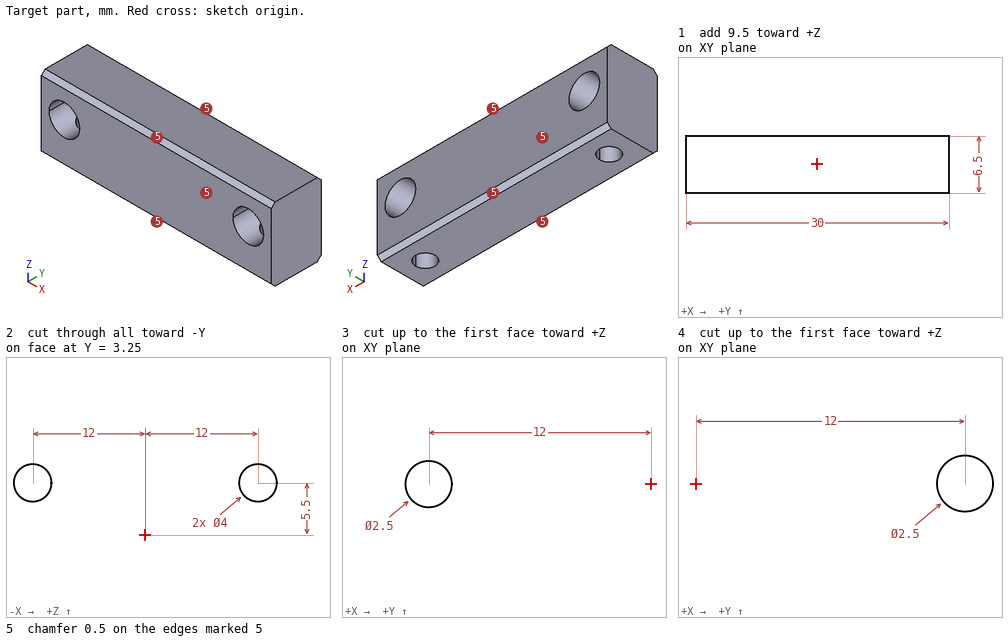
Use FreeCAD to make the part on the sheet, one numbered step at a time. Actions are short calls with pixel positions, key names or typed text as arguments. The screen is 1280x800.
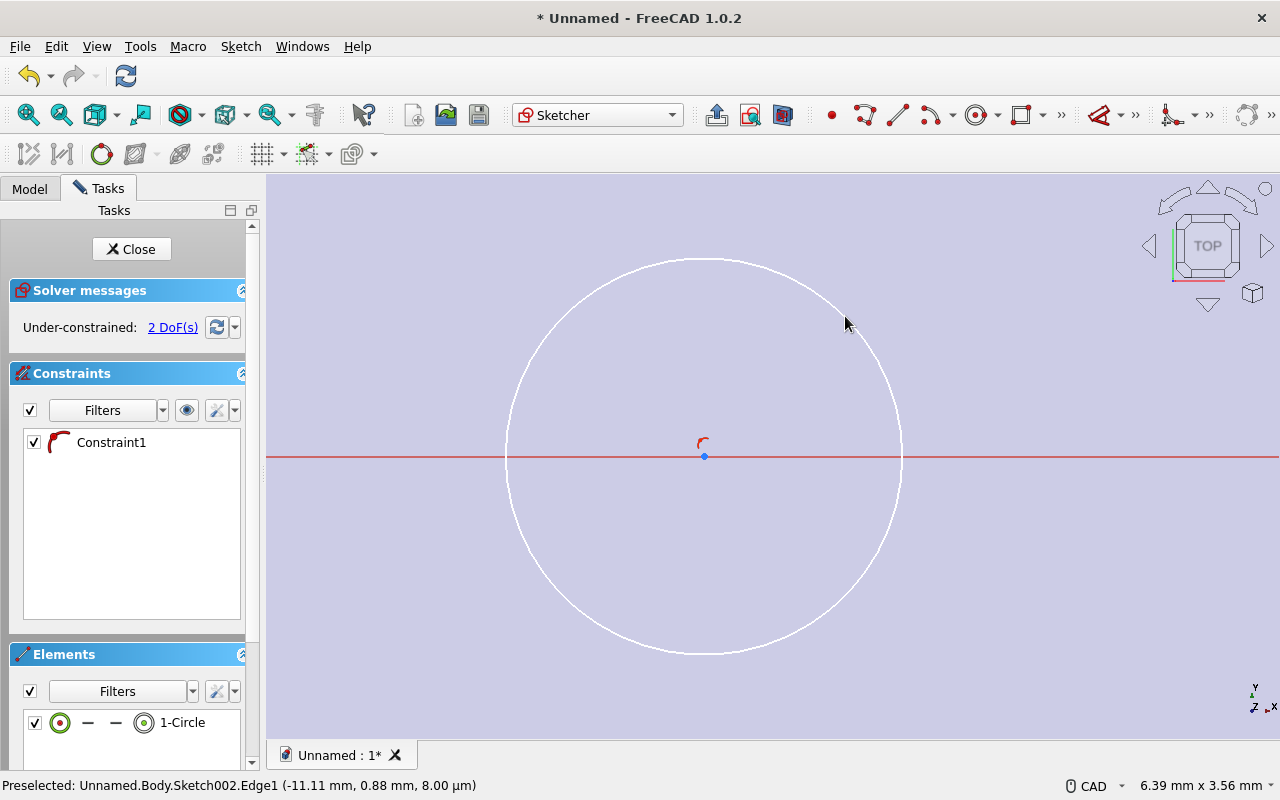
key(d)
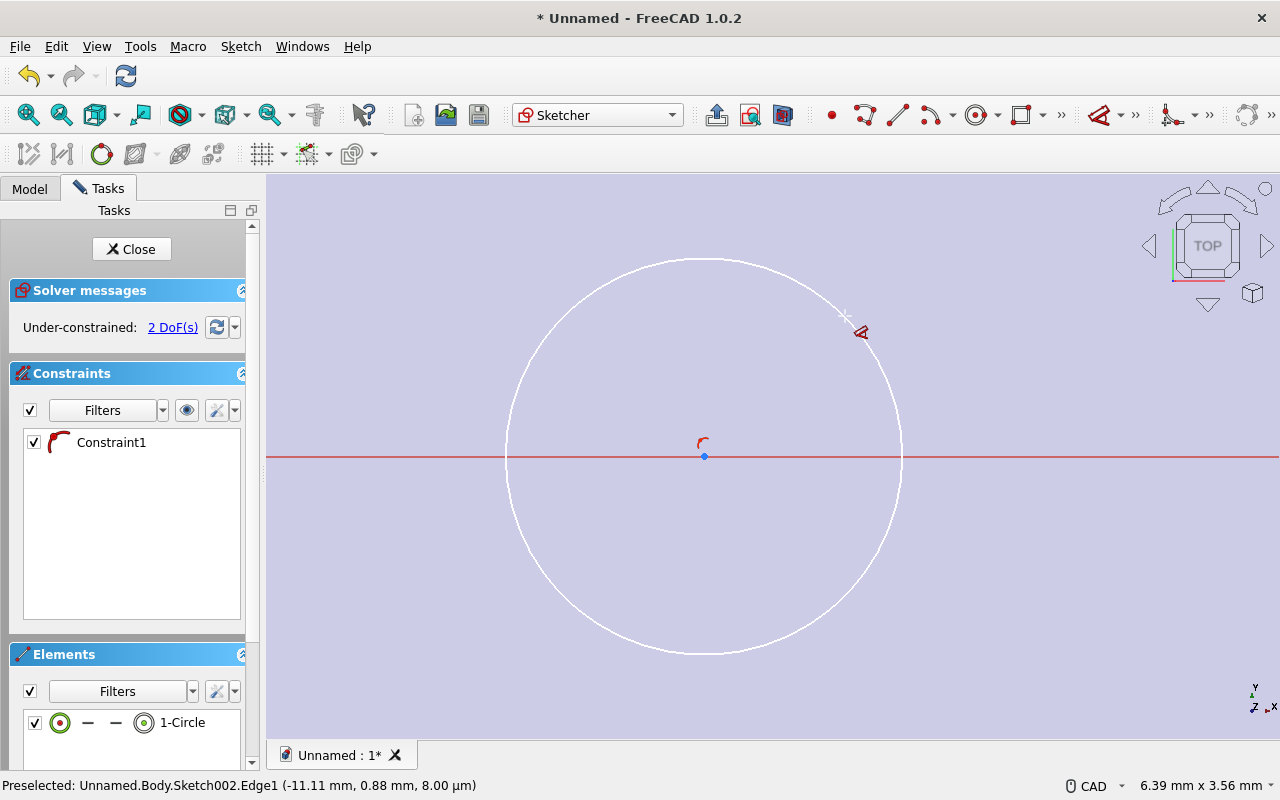
click(844, 316)
click(867, 293)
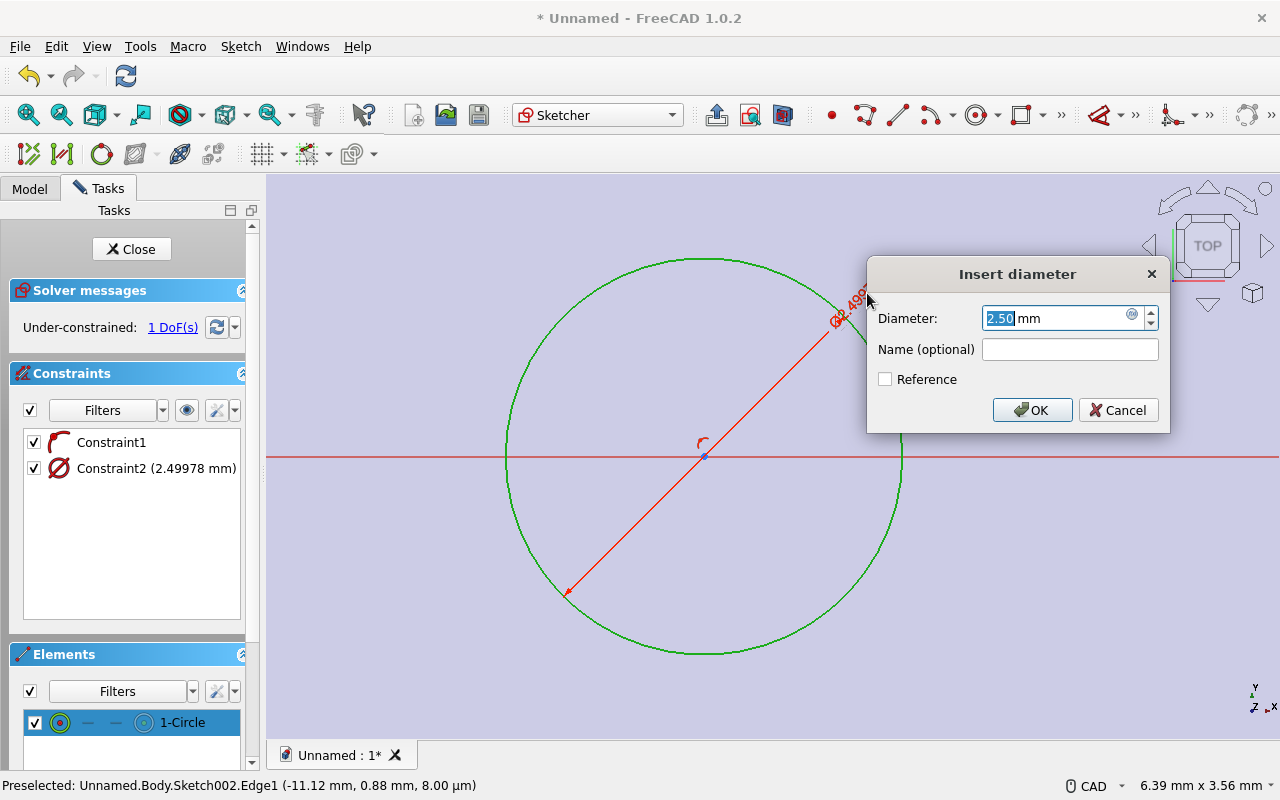
text(2.5)
key(Return)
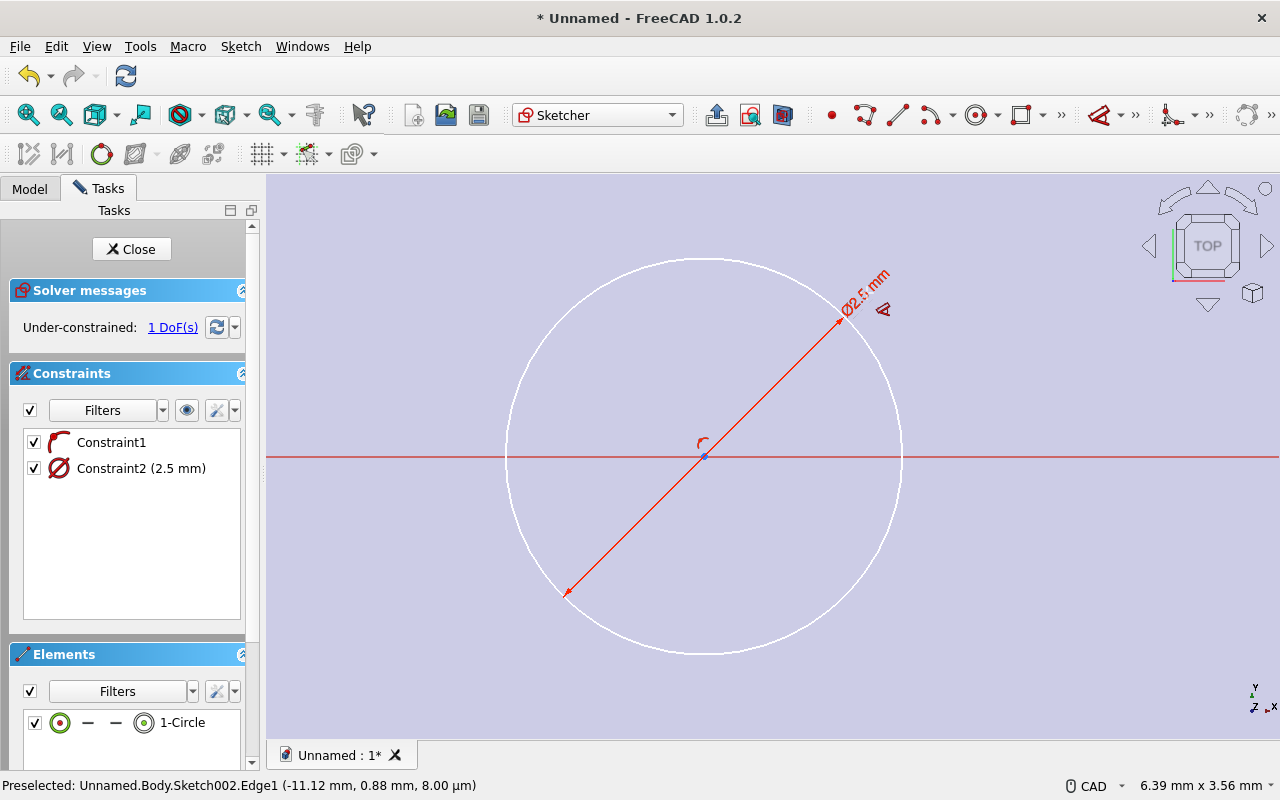
click(704, 456)
click(815, 490)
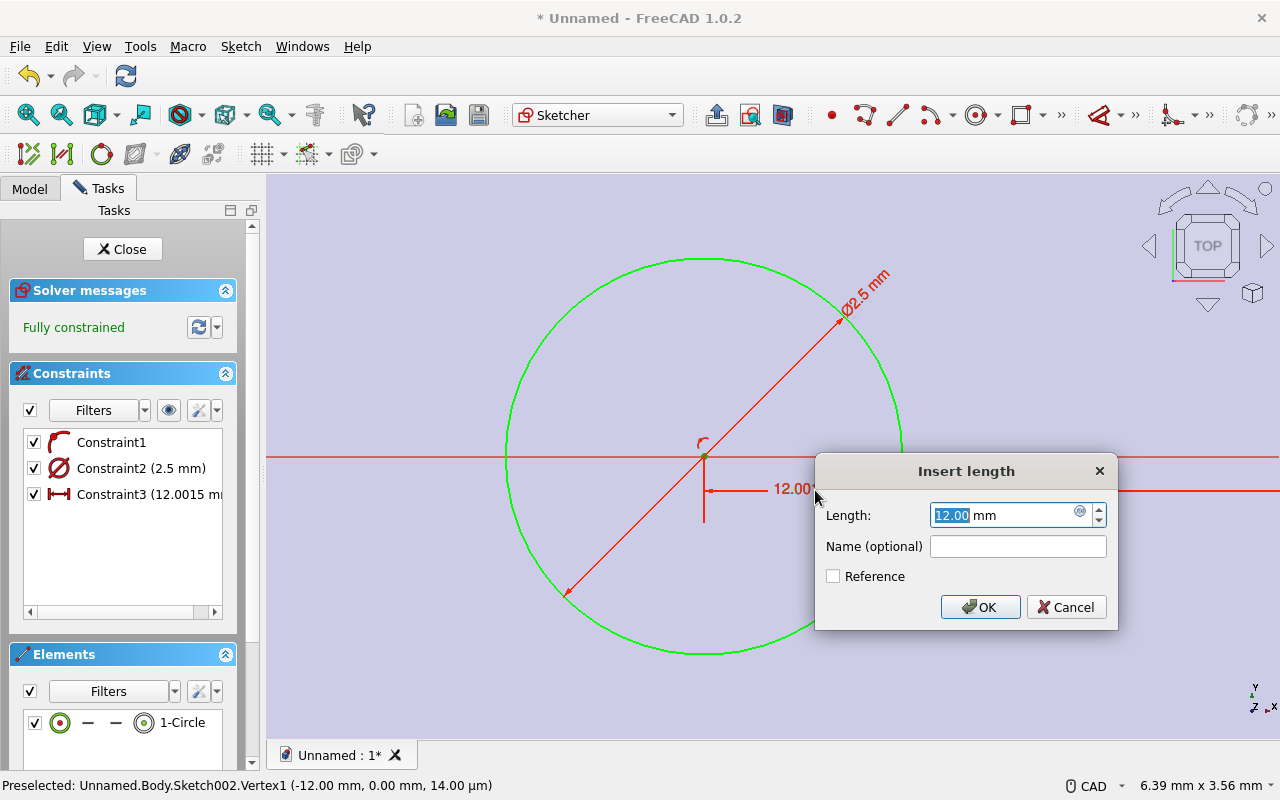
text(12)
key(Return)
key(Escape)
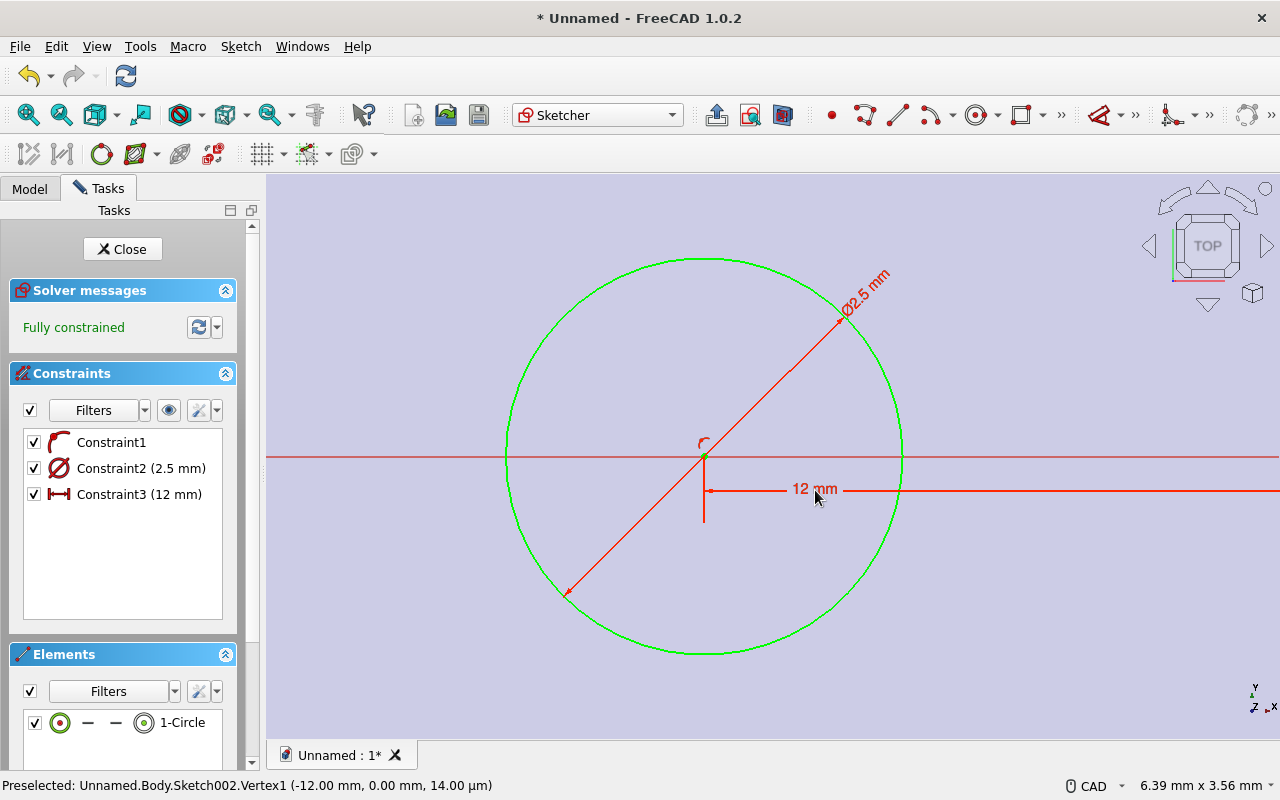
click(123, 249)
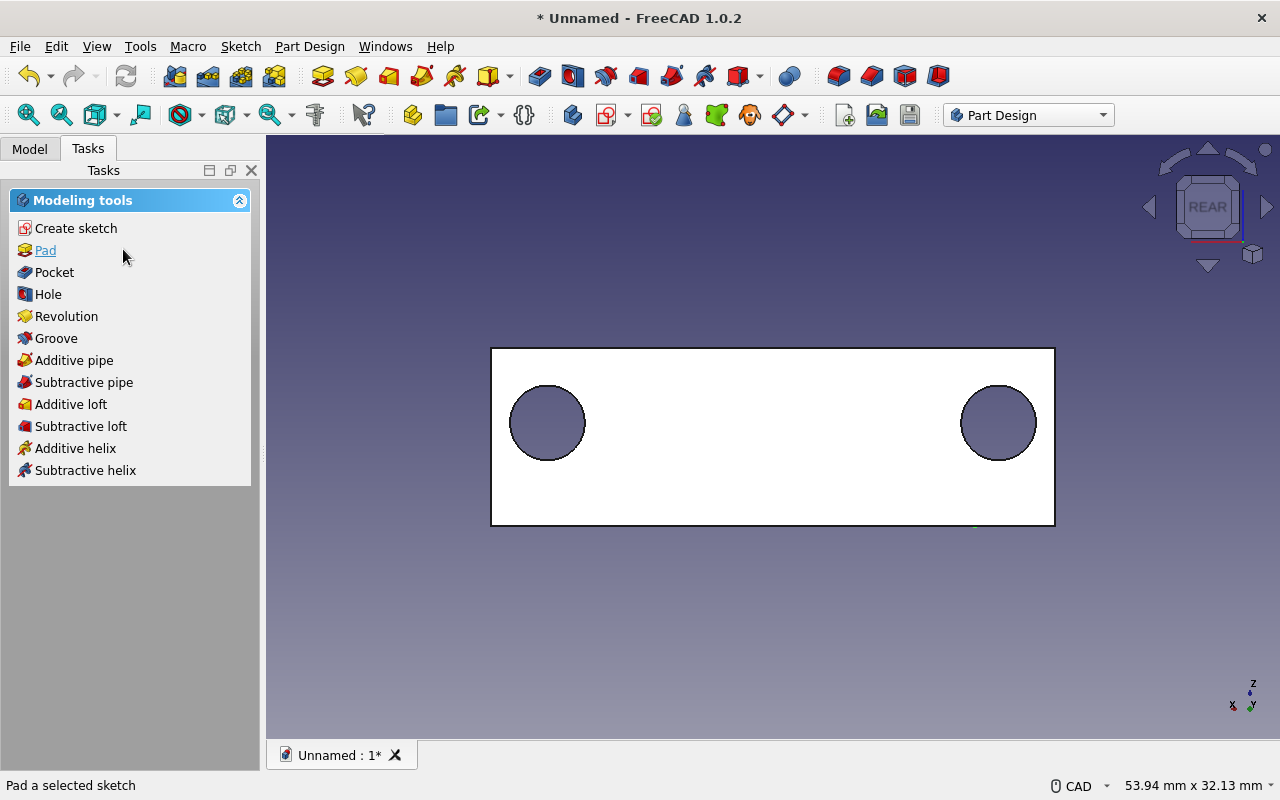
click(540, 76)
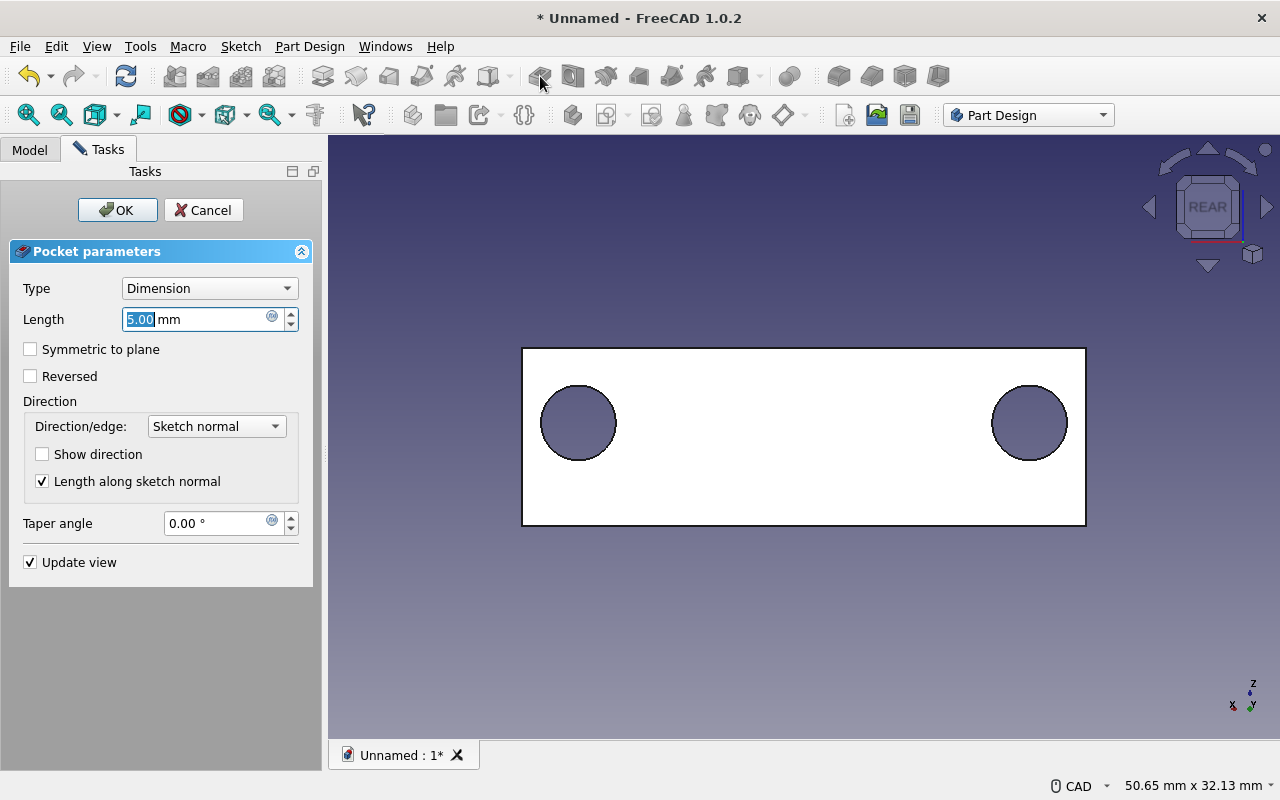
click(210, 288)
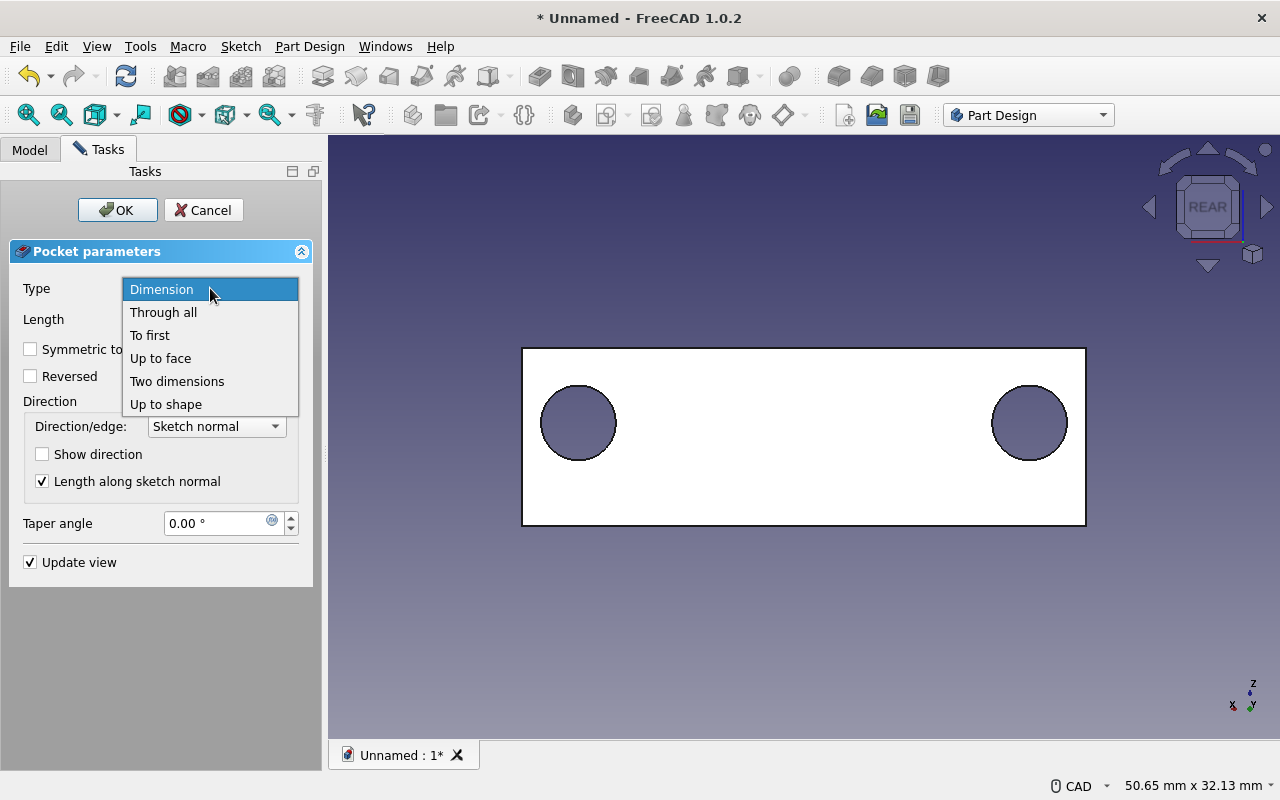
click(208, 336)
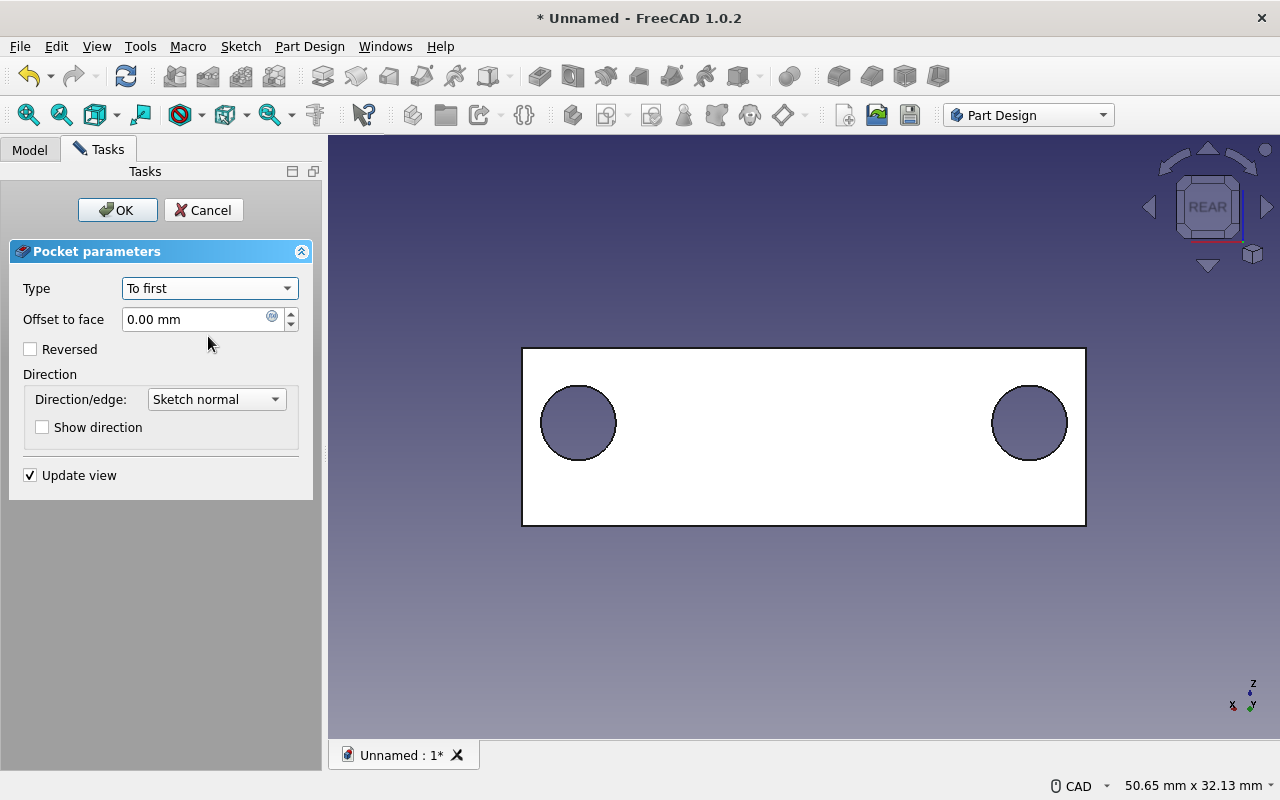
click(31, 349)